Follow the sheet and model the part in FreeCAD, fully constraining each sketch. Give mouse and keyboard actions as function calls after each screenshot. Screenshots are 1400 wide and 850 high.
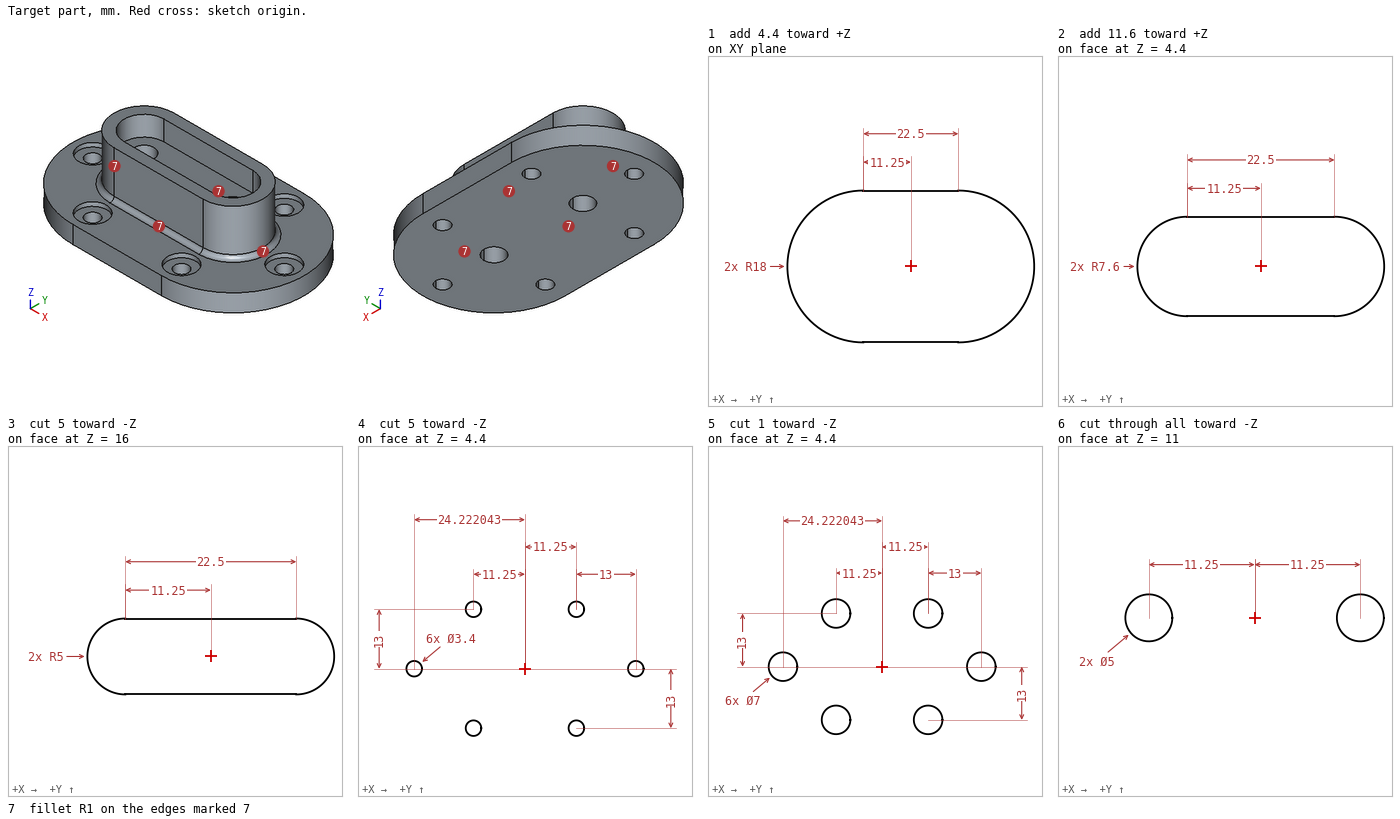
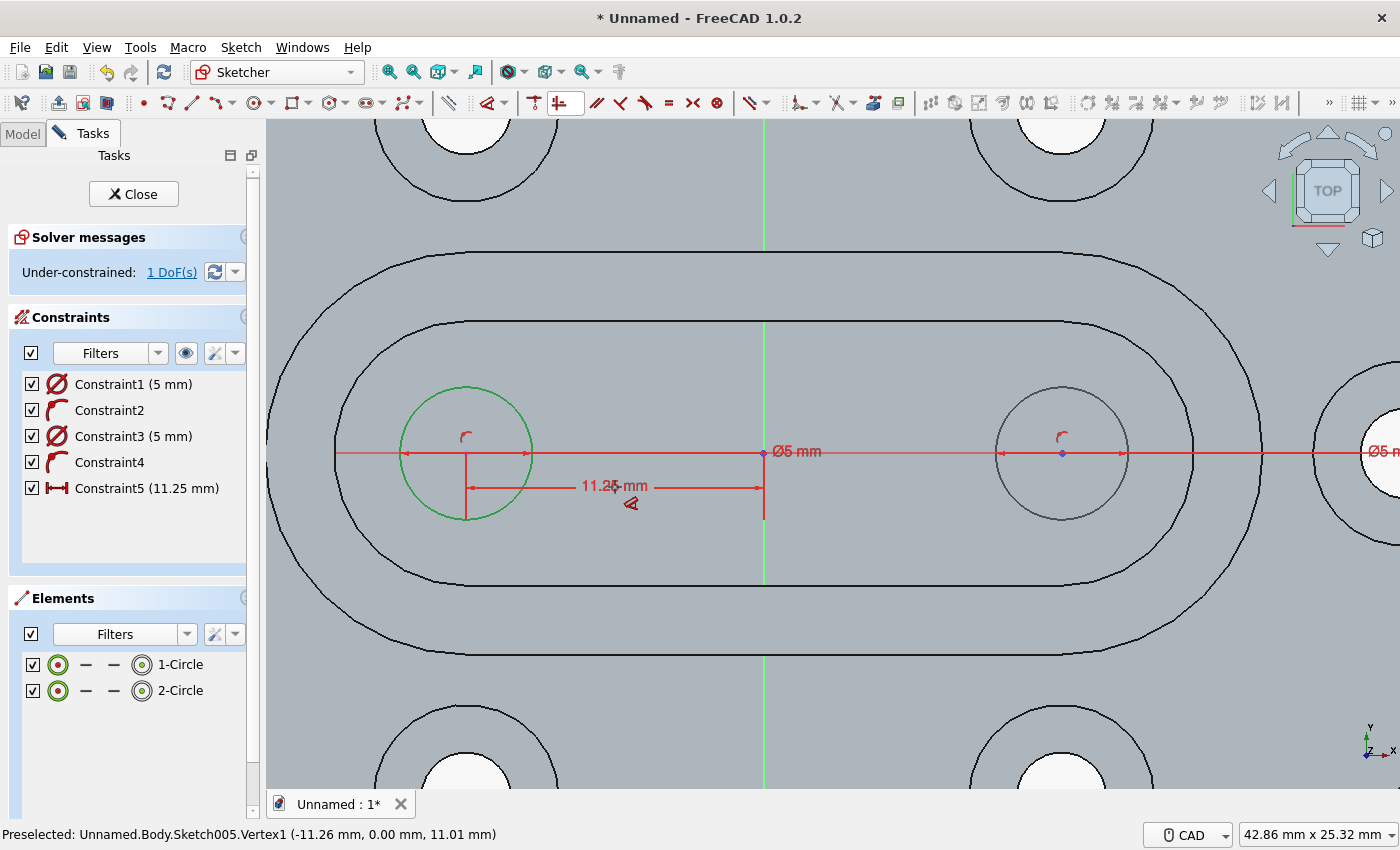
click(1062, 453)
click(913, 487)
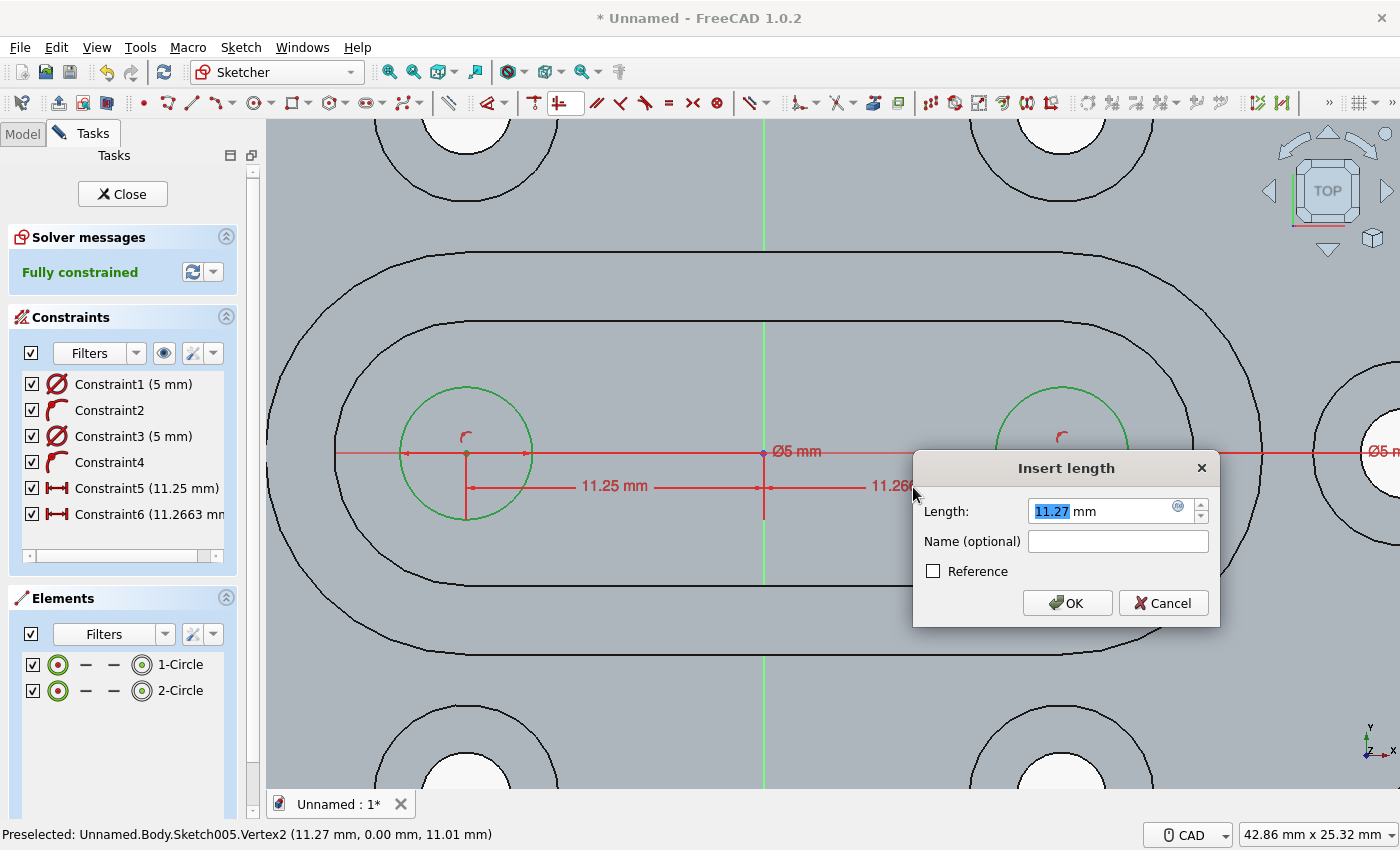
text(11.25)
key(Return)
key(Escape)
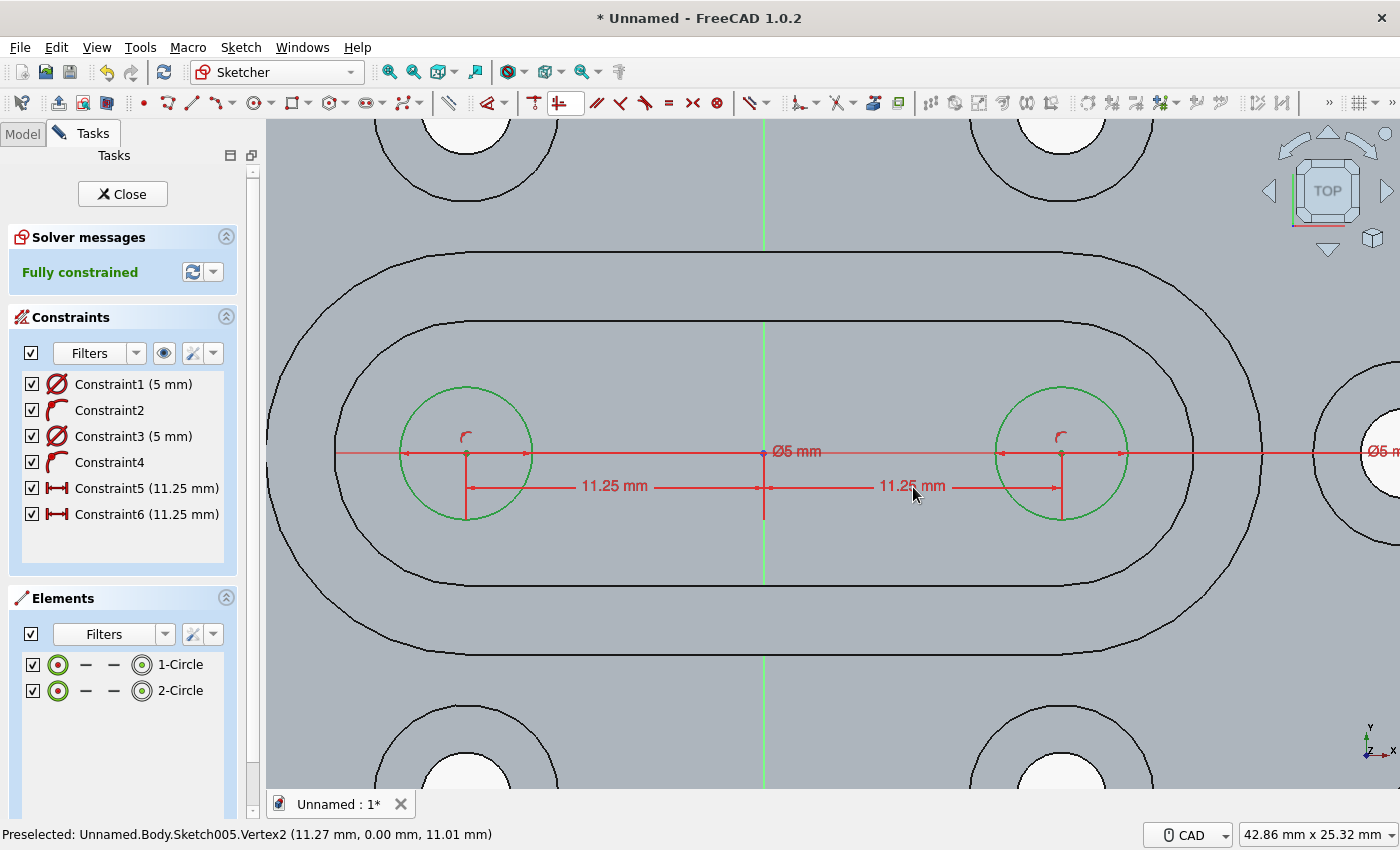
click(123, 194)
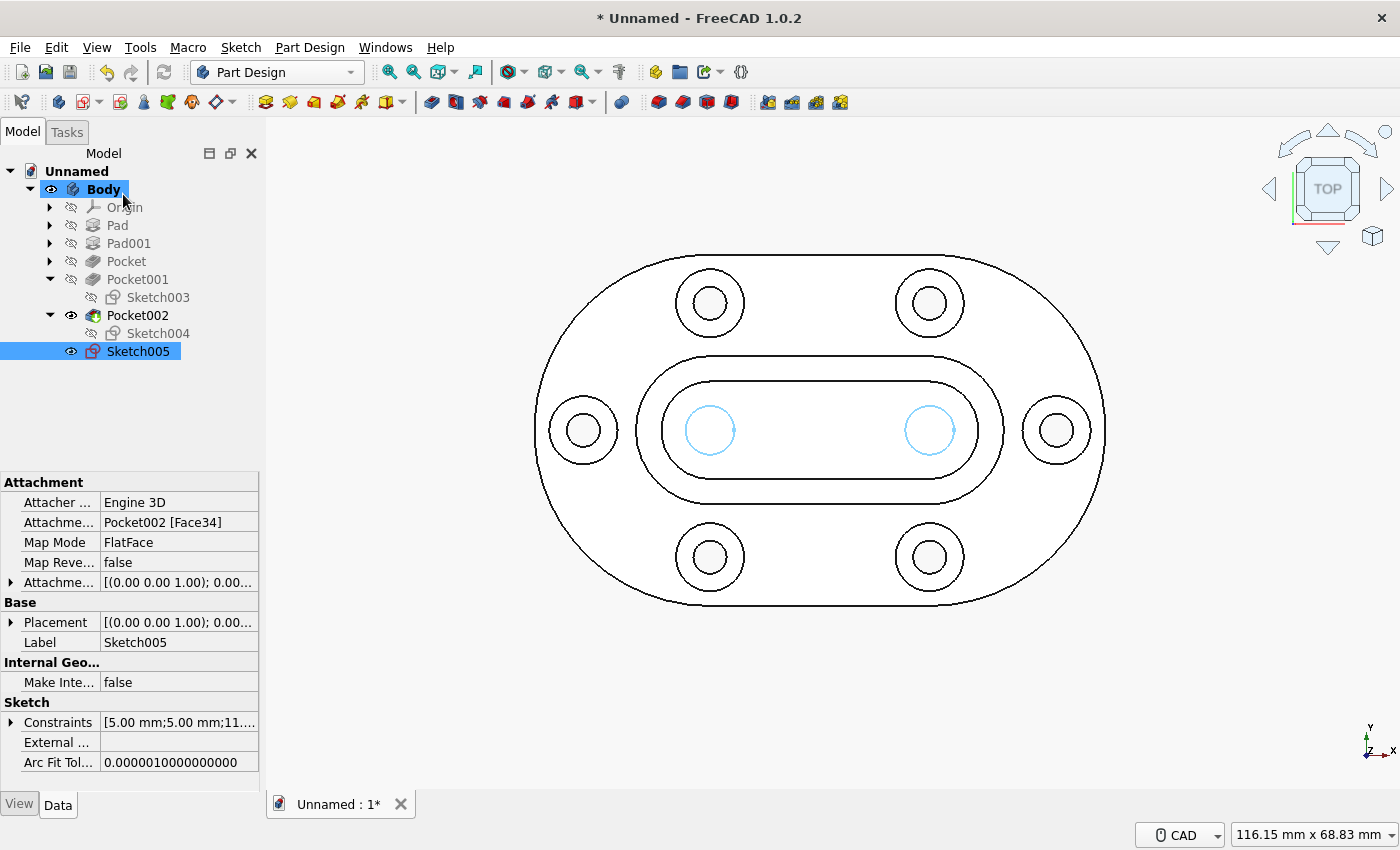
click(432, 102)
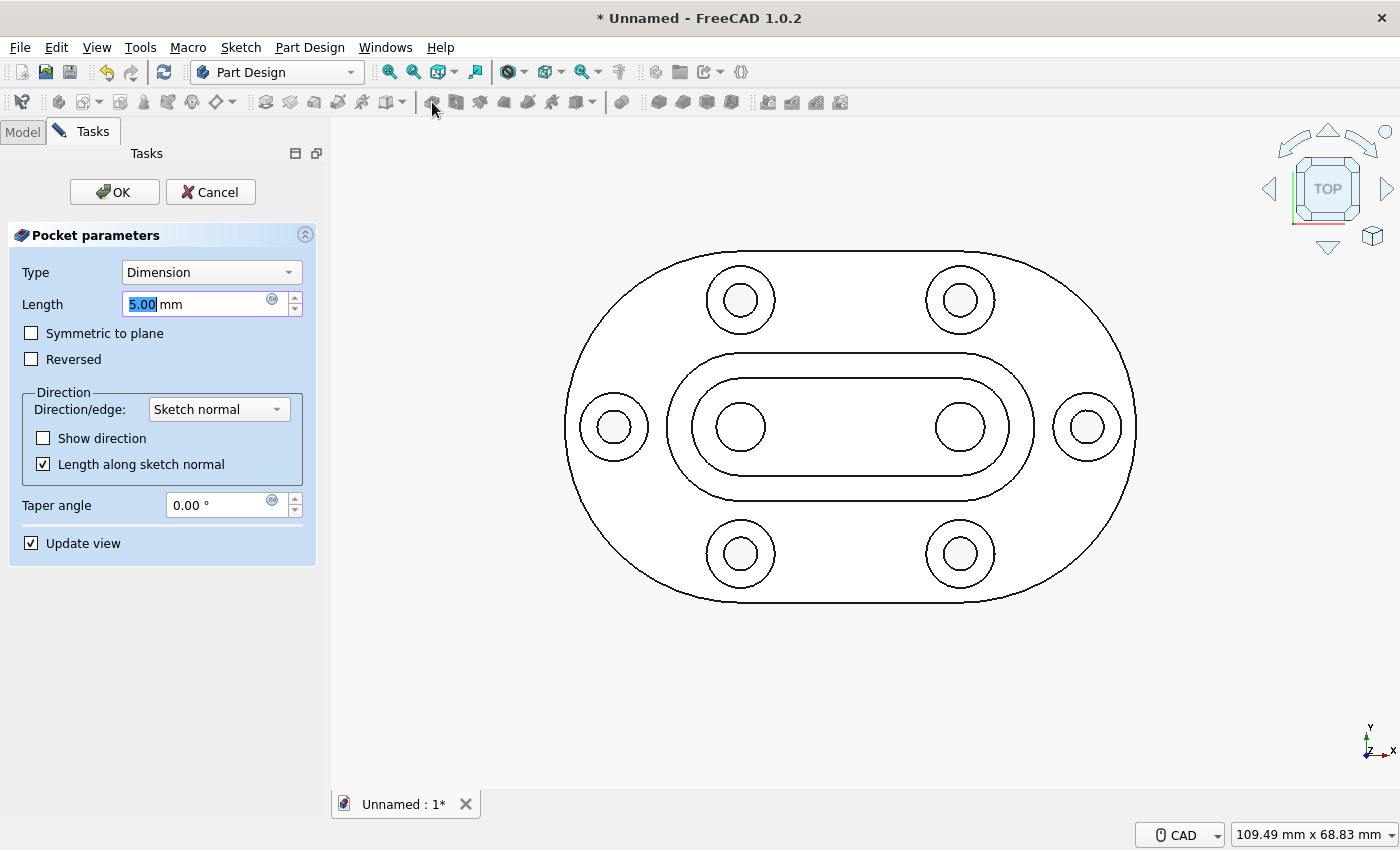
click(212, 272)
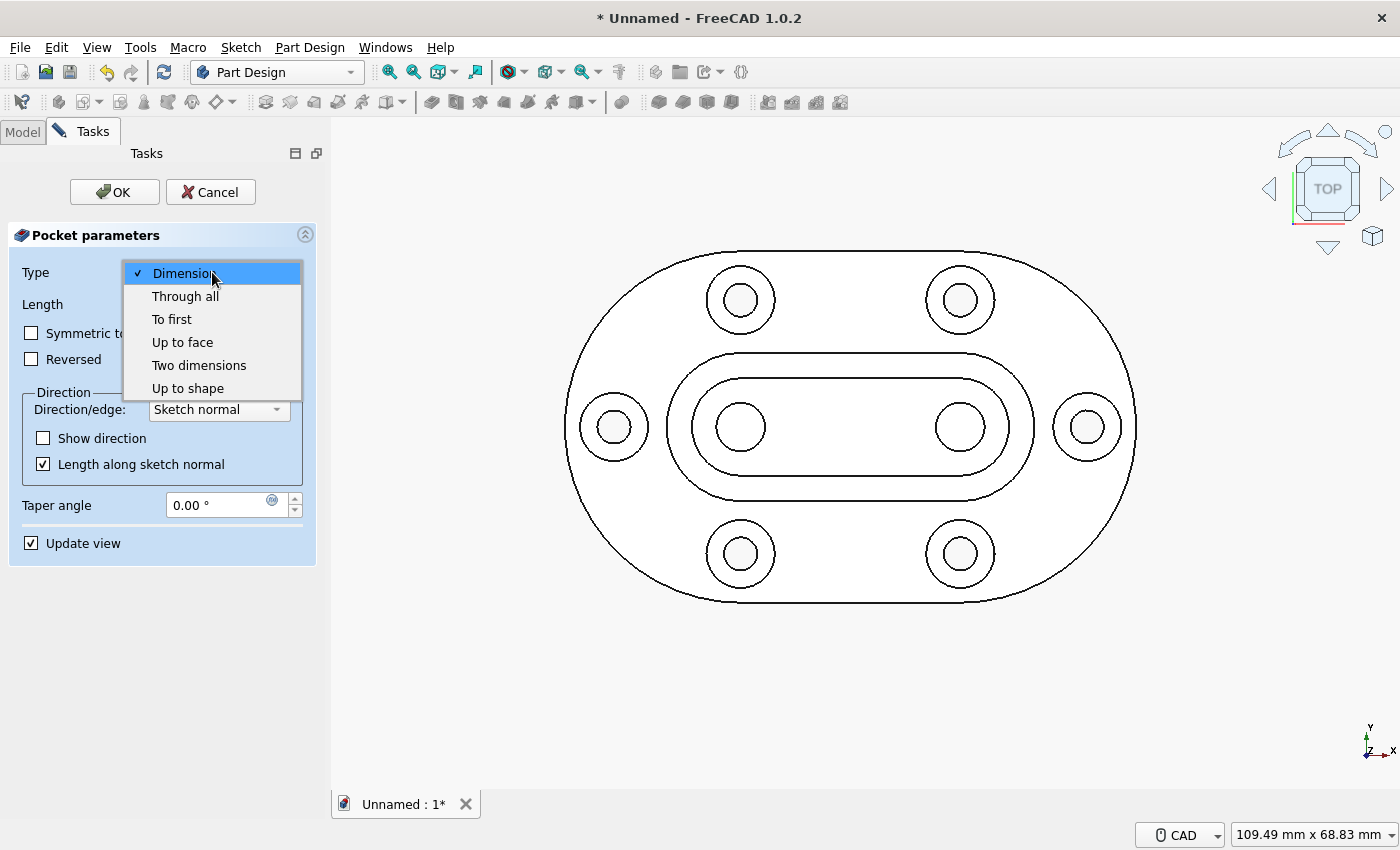
click(212, 296)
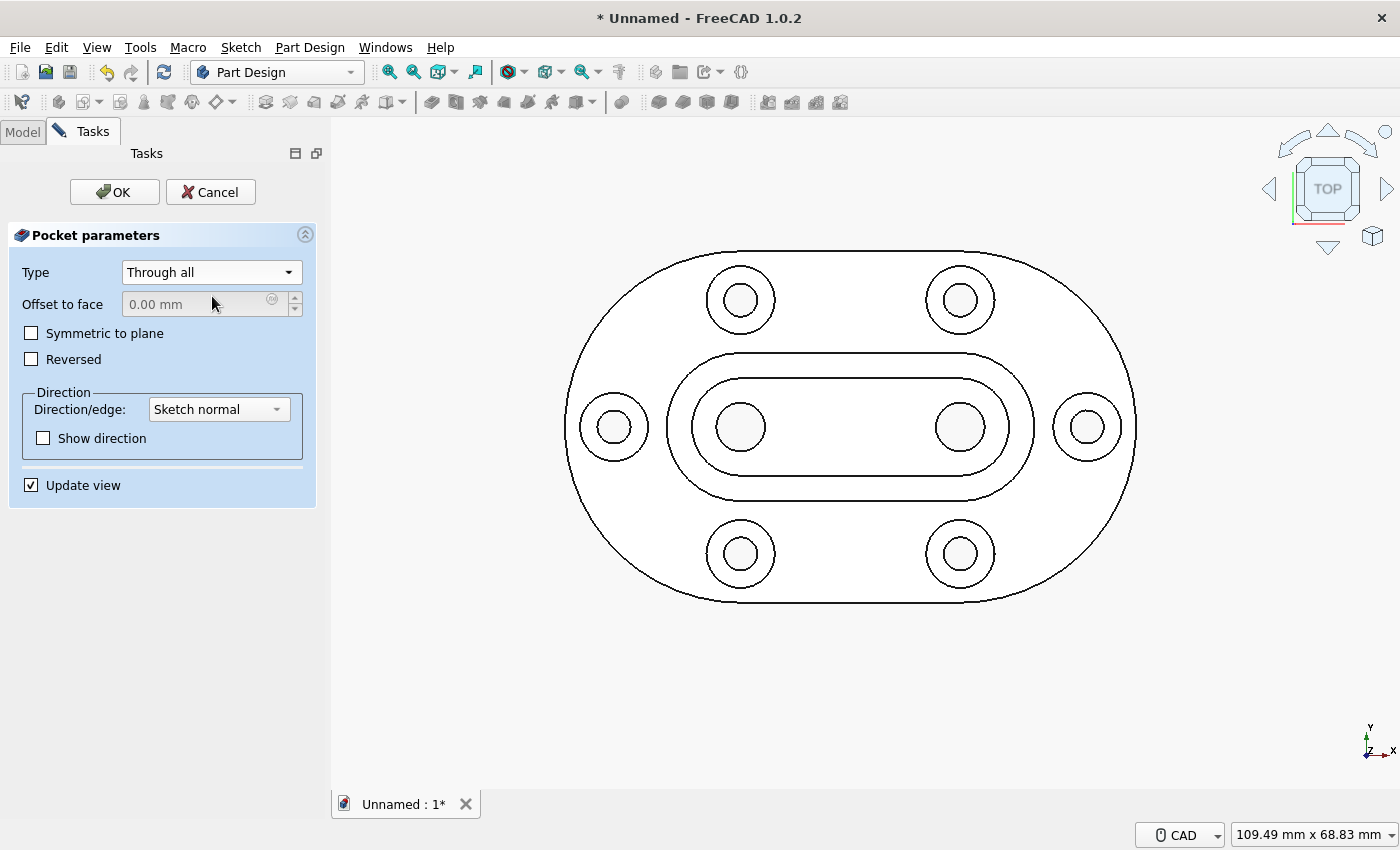
click(115, 192)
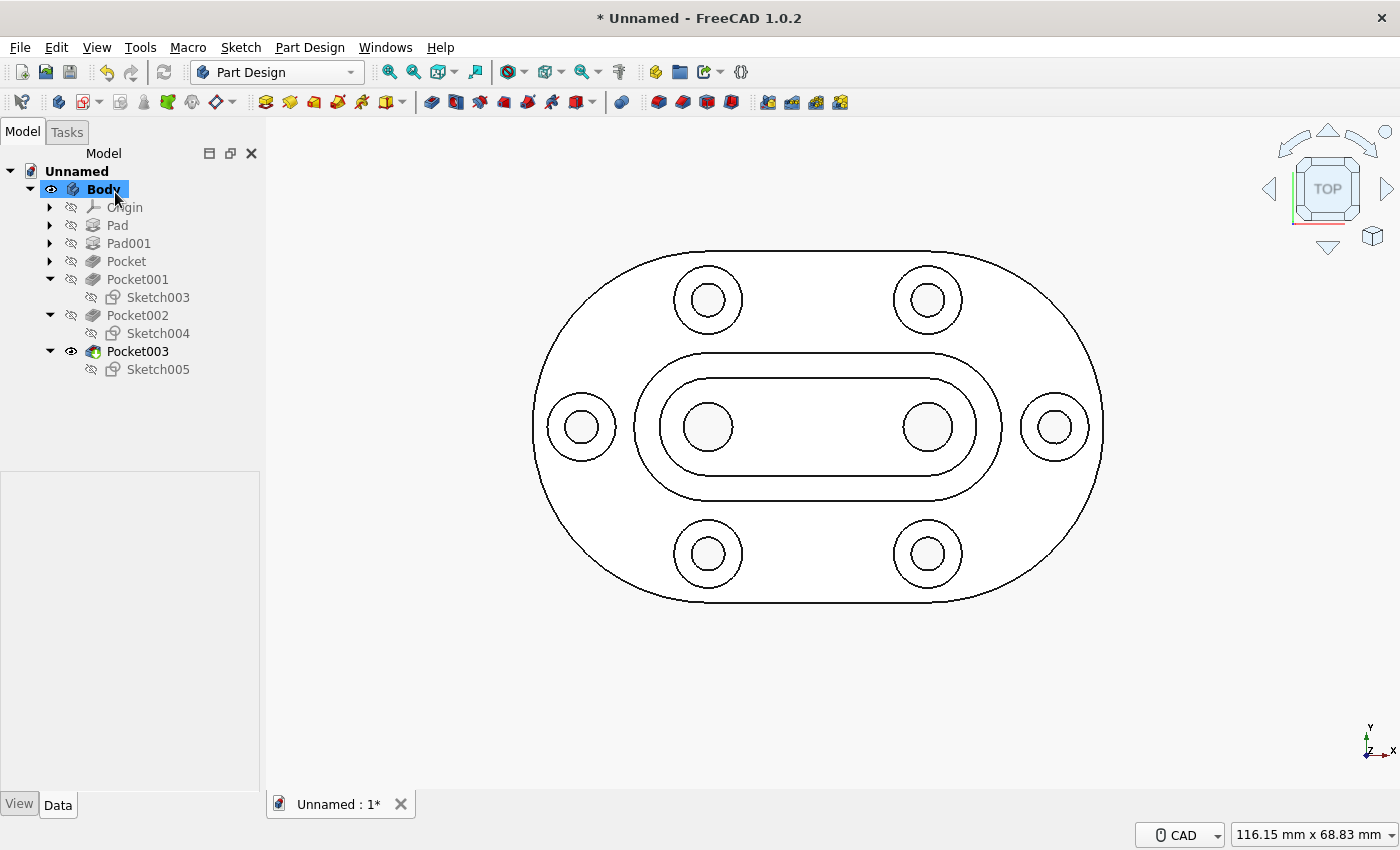
key(0)